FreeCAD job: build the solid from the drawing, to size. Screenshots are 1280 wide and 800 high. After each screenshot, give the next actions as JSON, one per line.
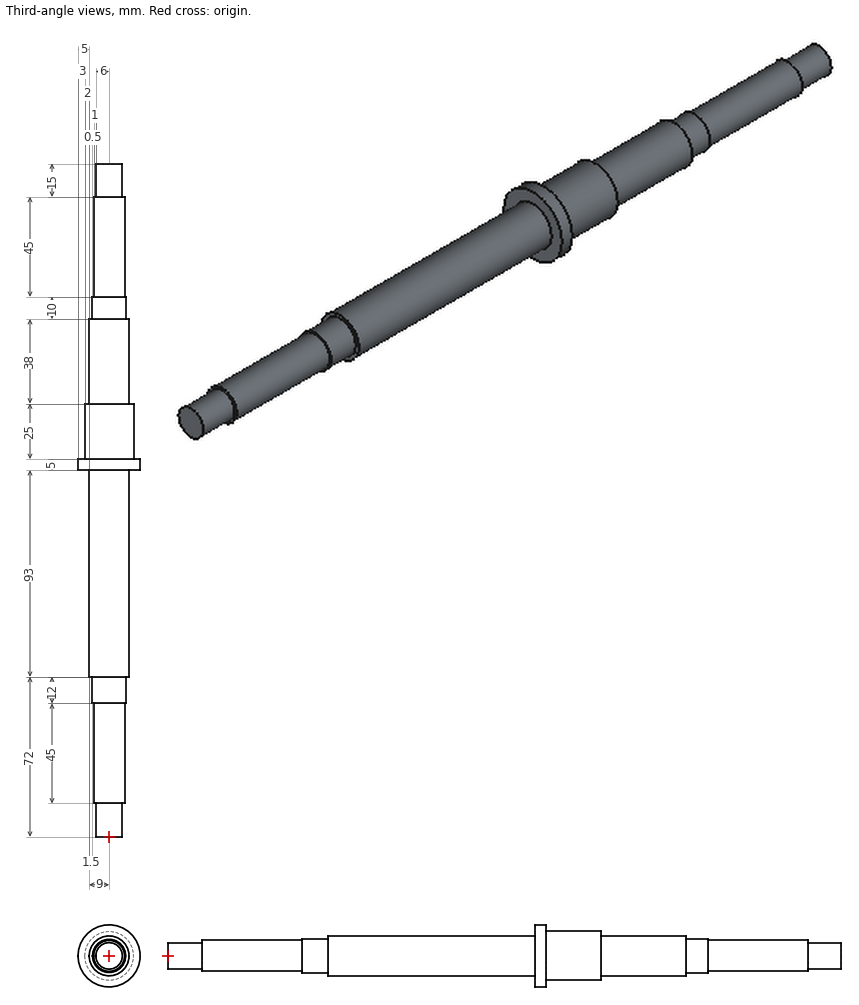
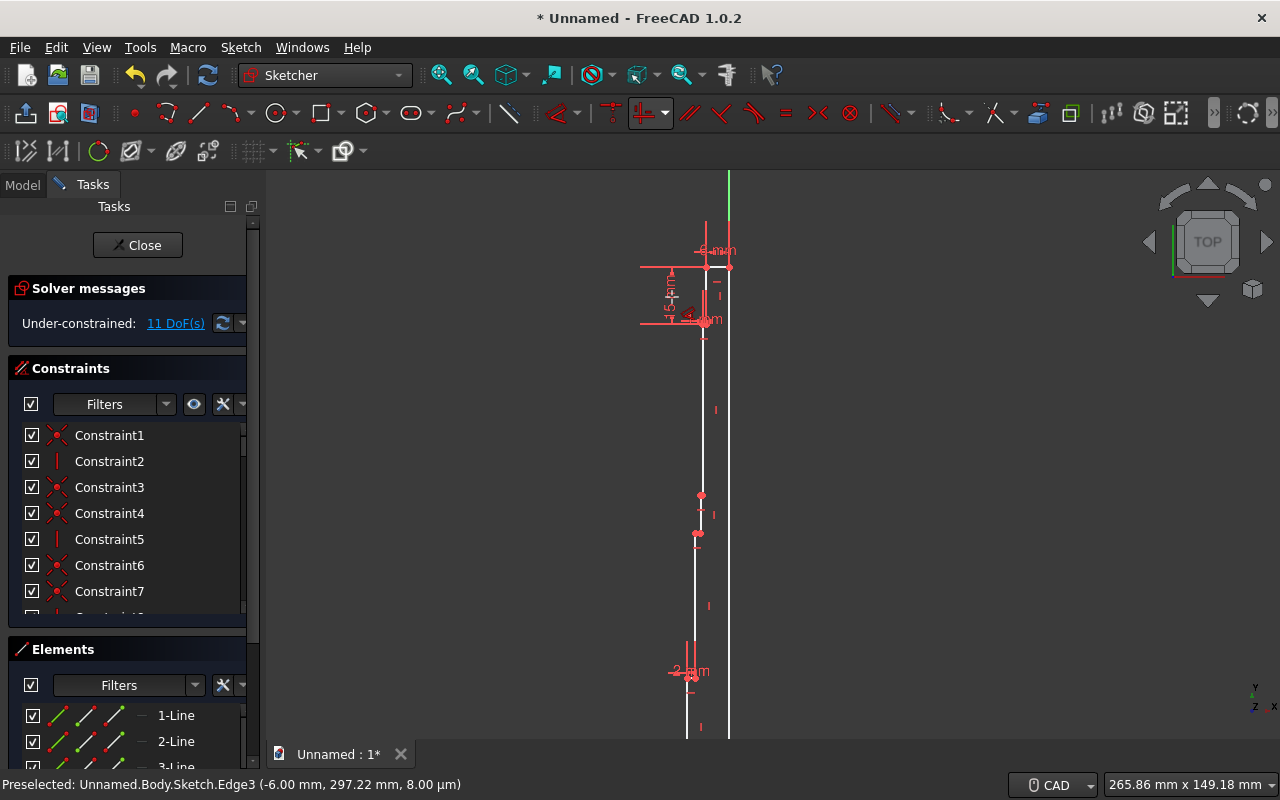
{"action": "left_click", "coordinate": [703, 376]}
{"action": "left_click", "coordinate": [669, 410]}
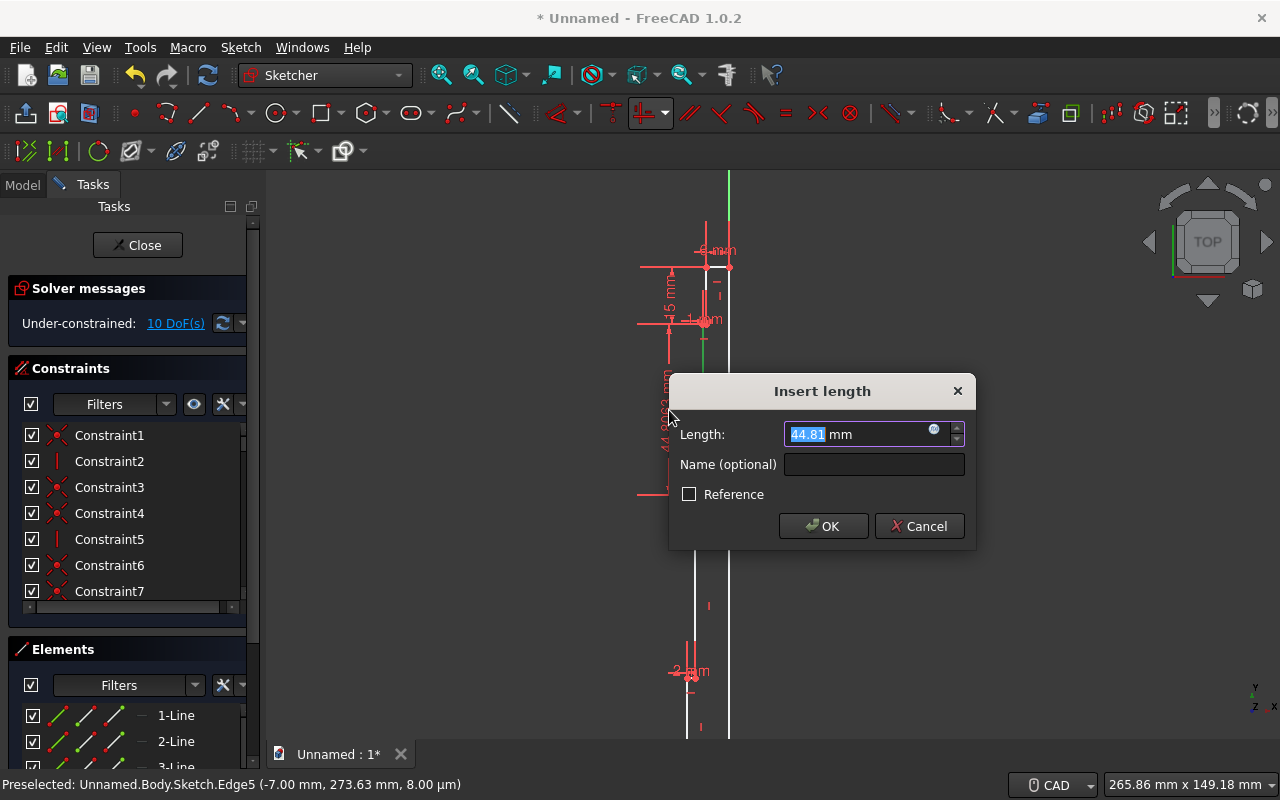
{"action": "type", "text": "45"}
{"action": "key", "text": "Return"}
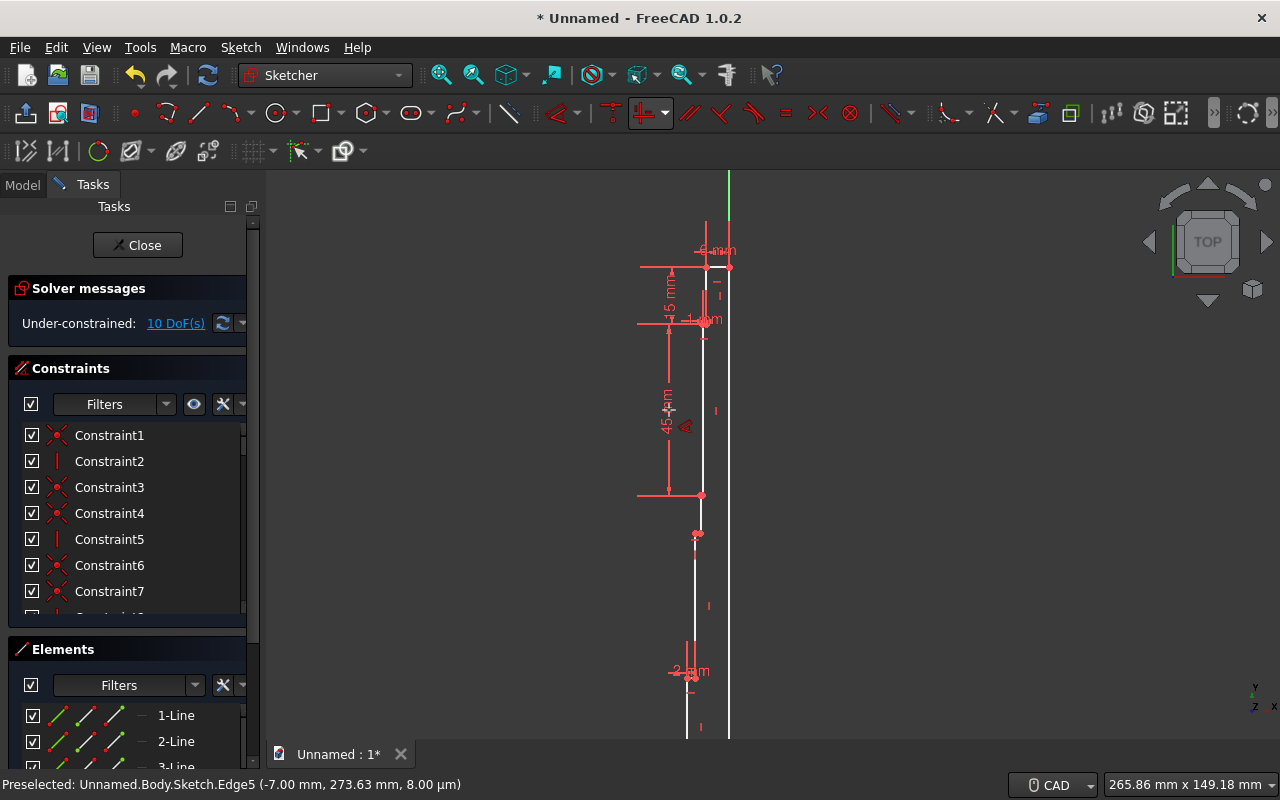
{"action": "scroll", "coordinate": [701, 507], "scroll_direction": "up", "scroll_amount": 2}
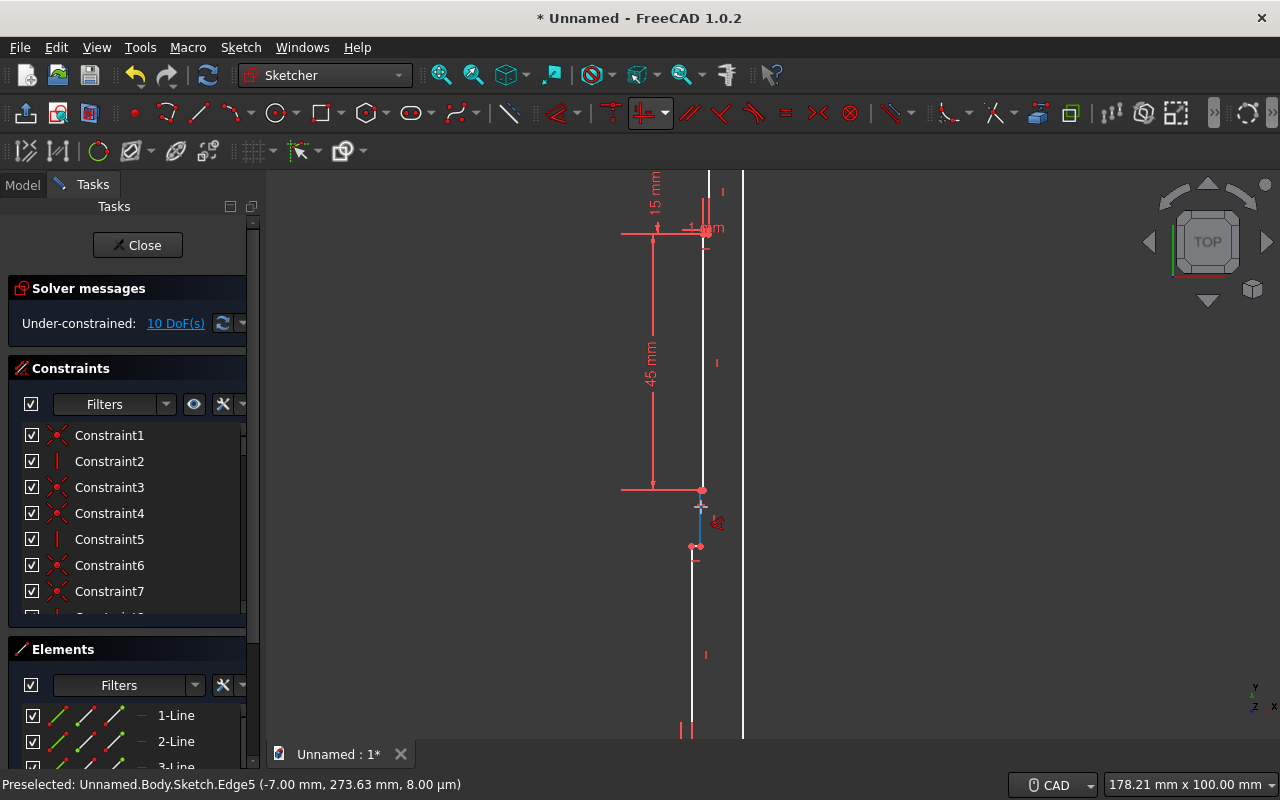
{"action": "left_click", "coordinate": [700, 507]}
{"action": "left_click", "coordinate": [666, 518]}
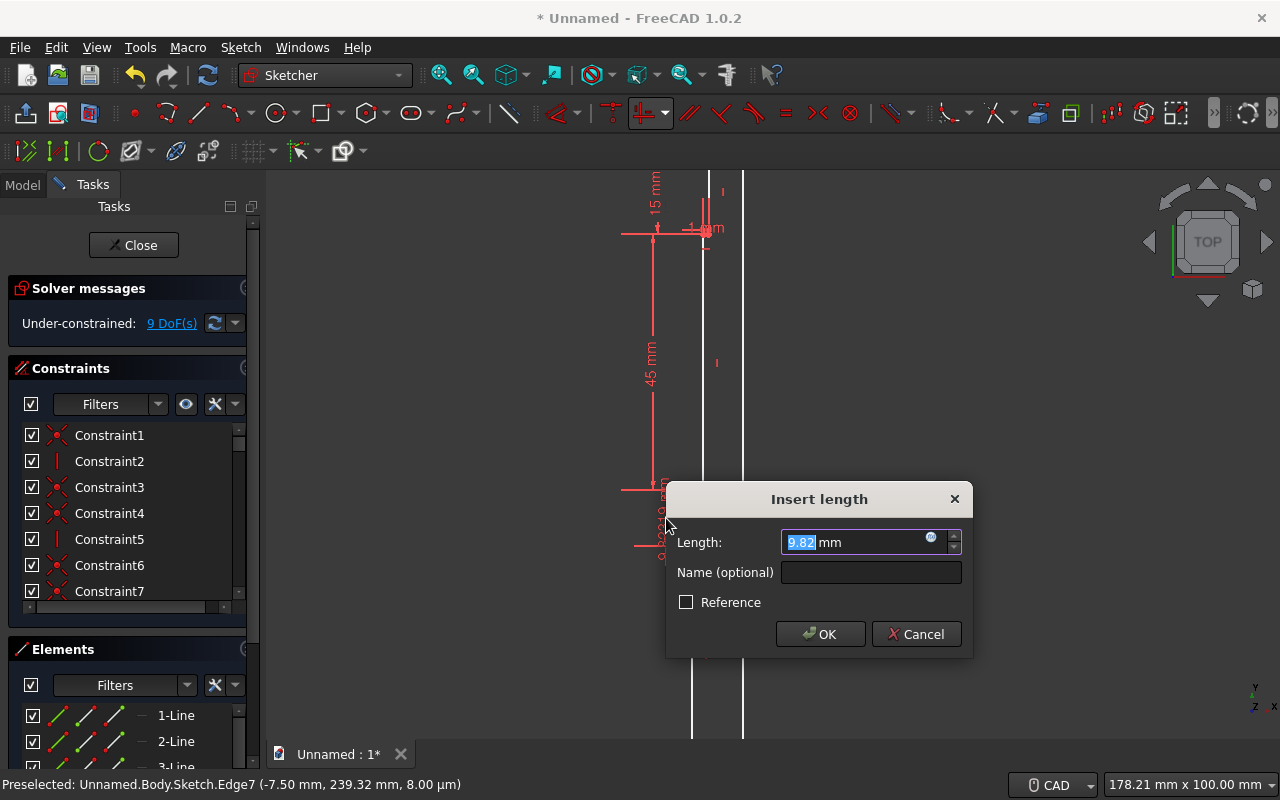
{"action": "type", "text": "10"}
{"action": "key", "text": "Return"}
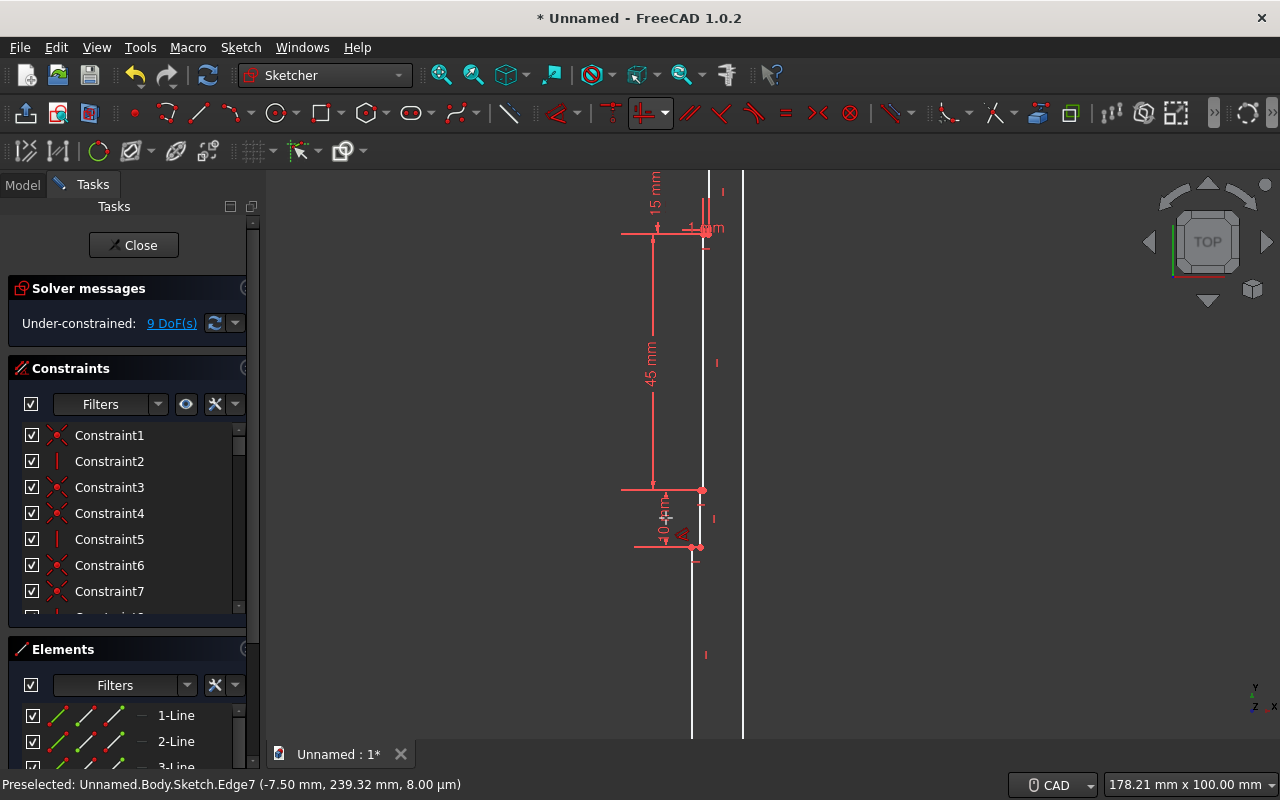
{"action": "scroll", "coordinate": [705, 315], "scroll_direction": "down", "scroll_amount": 8}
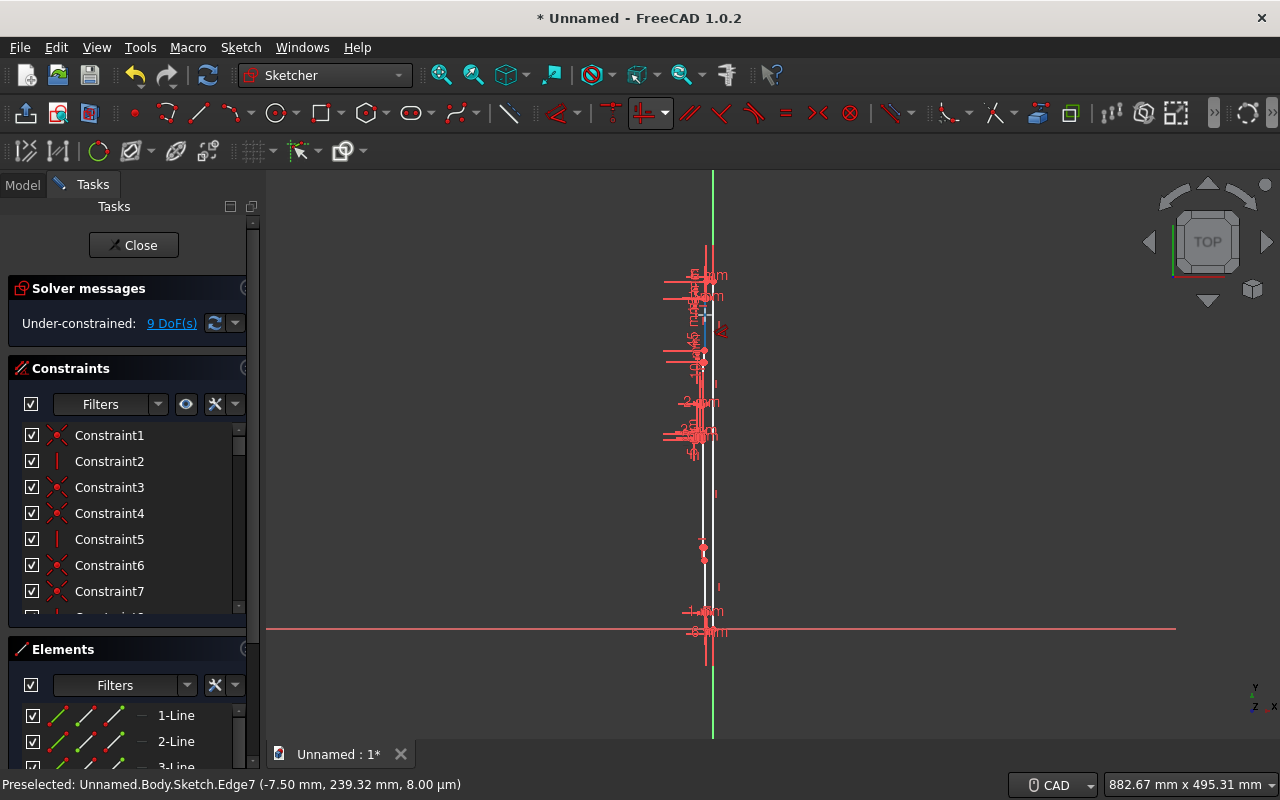
{"action": "scroll", "coordinate": [703, 375], "scroll_direction": "up", "scroll_amount": 2}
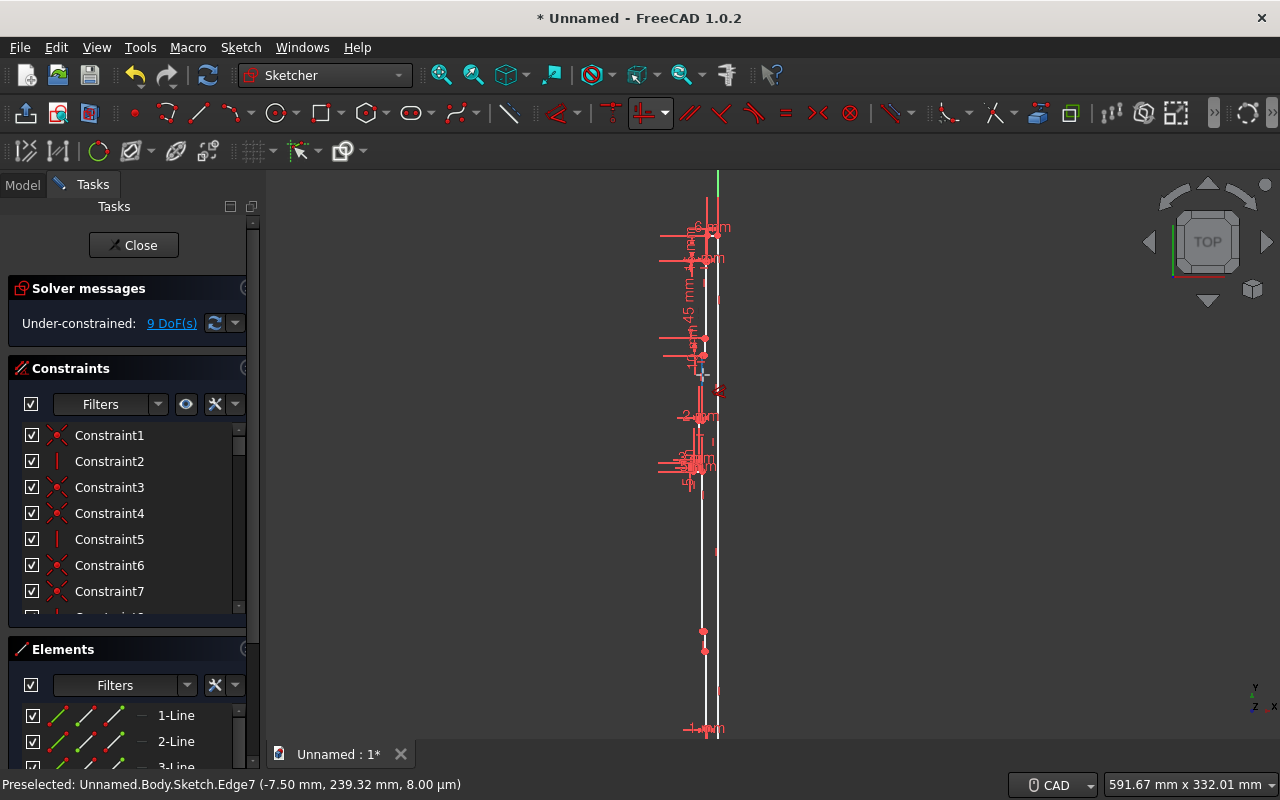
{"action": "left_click", "coordinate": [702, 375]}
{"action": "left_click", "coordinate": [668, 388]}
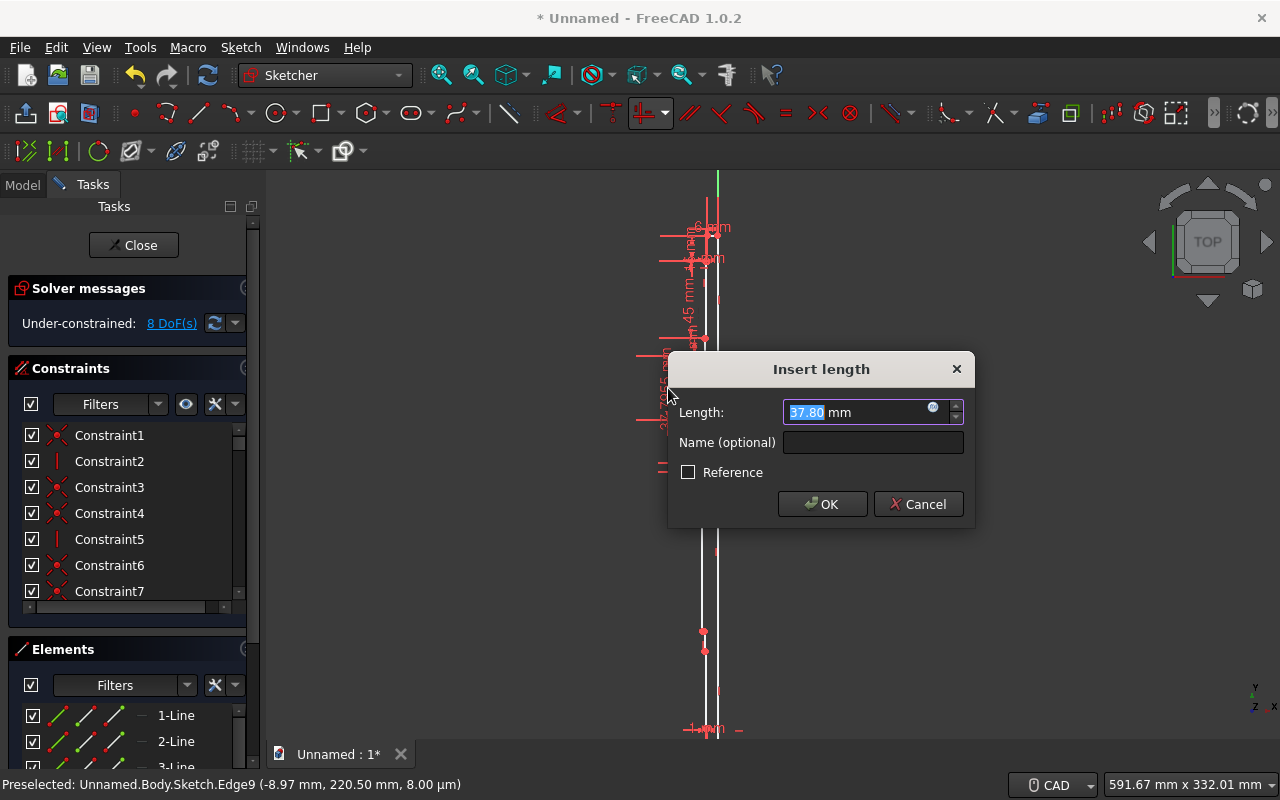
{"action": "type", "text": "38"}
{"action": "key", "text": "Return"}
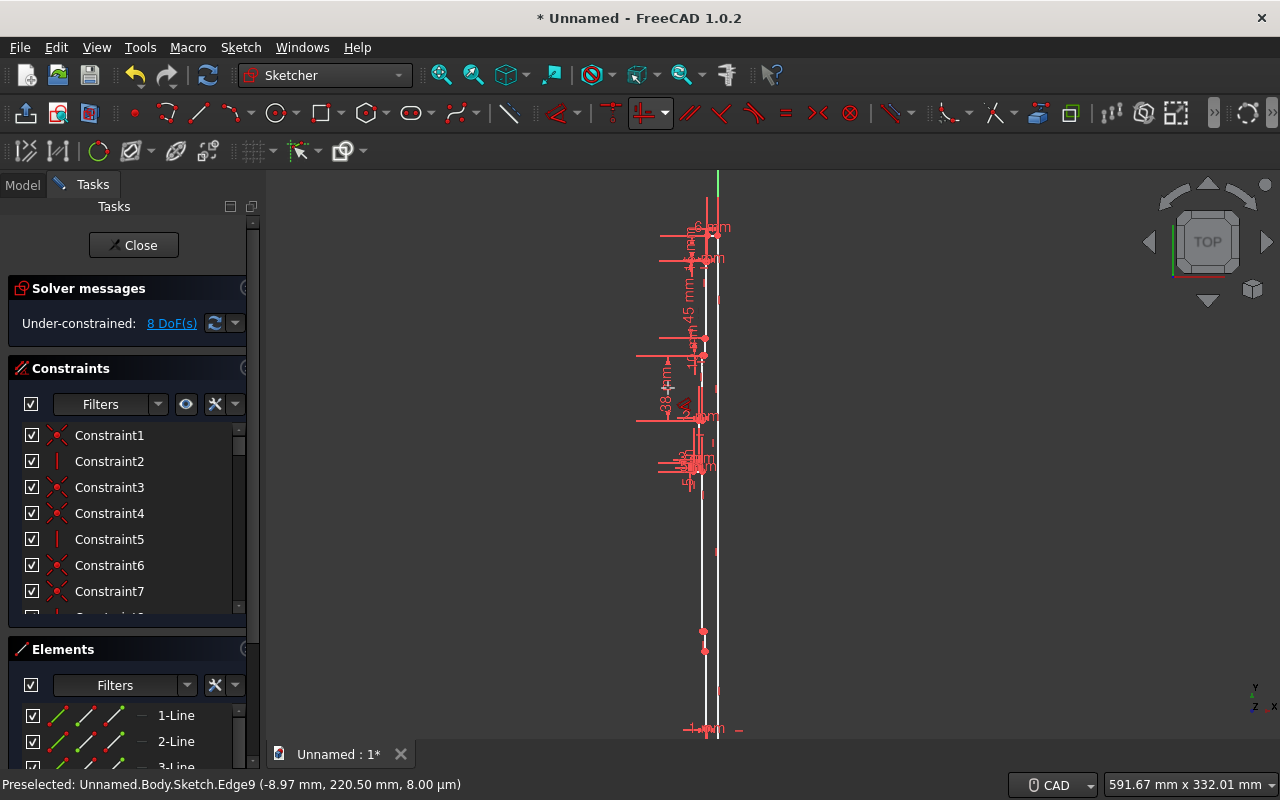
{"action": "left_click", "coordinate": [699, 433]}
{"action": "left_click", "coordinate": [617, 442]}